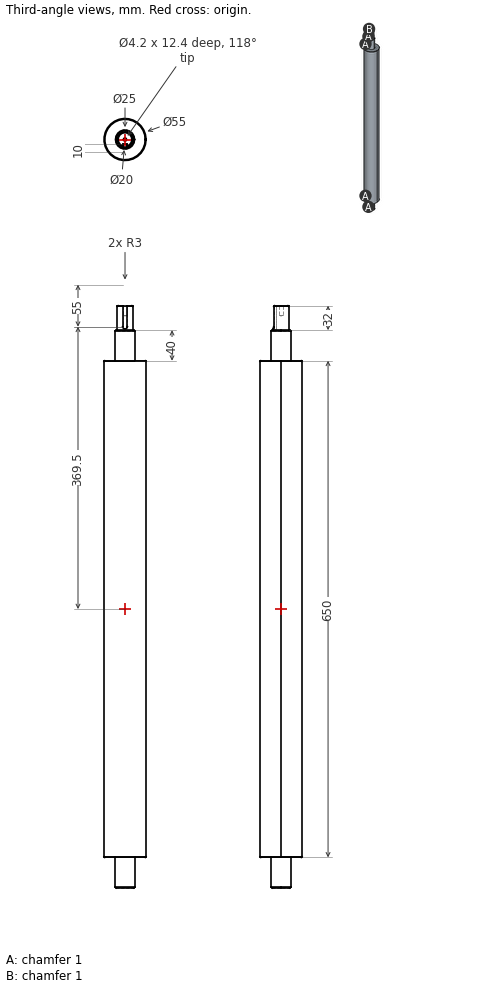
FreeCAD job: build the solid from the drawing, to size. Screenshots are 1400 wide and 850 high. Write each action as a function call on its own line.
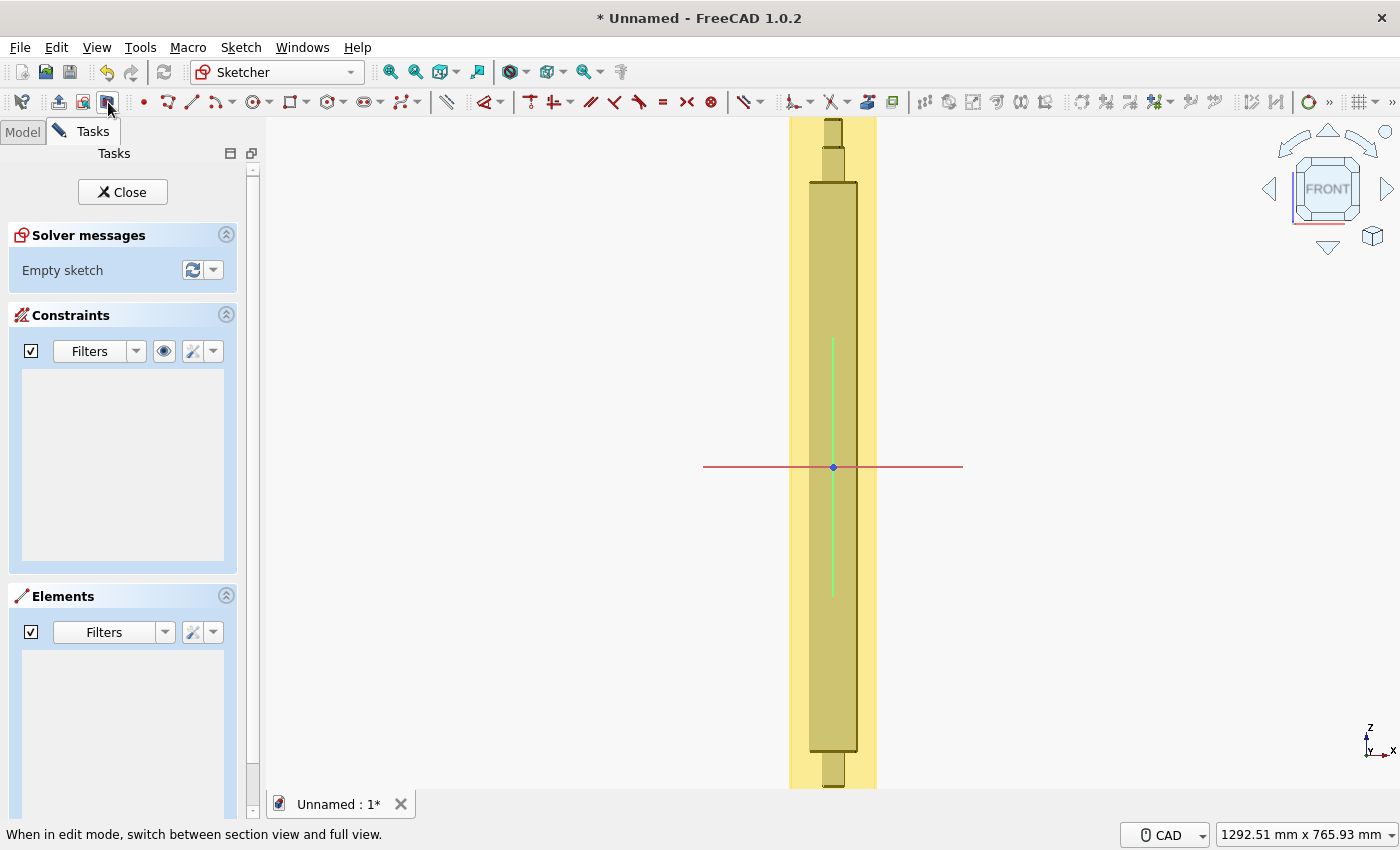
scroll(764, 453, down, 5)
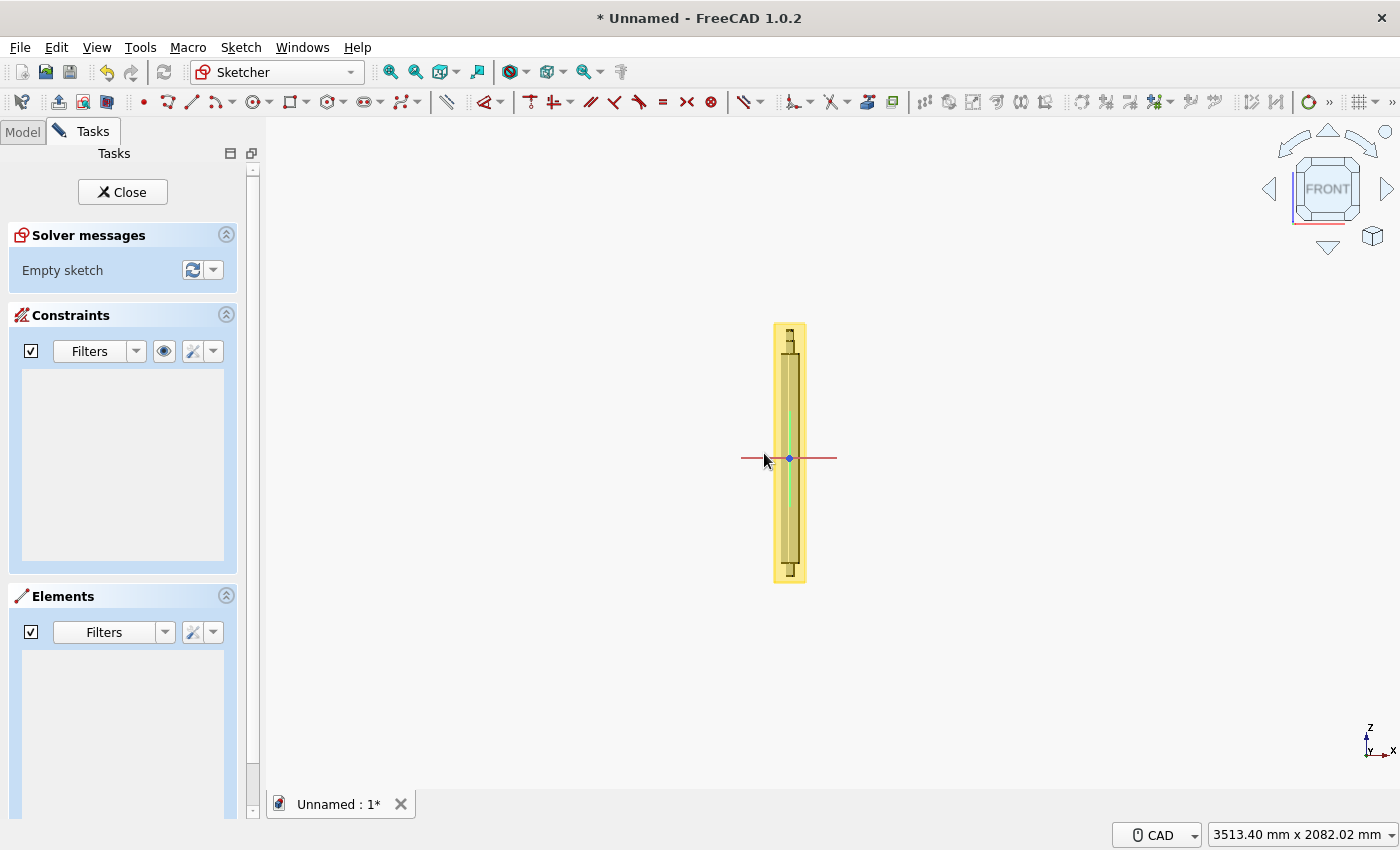
scroll(791, 324, up, 15)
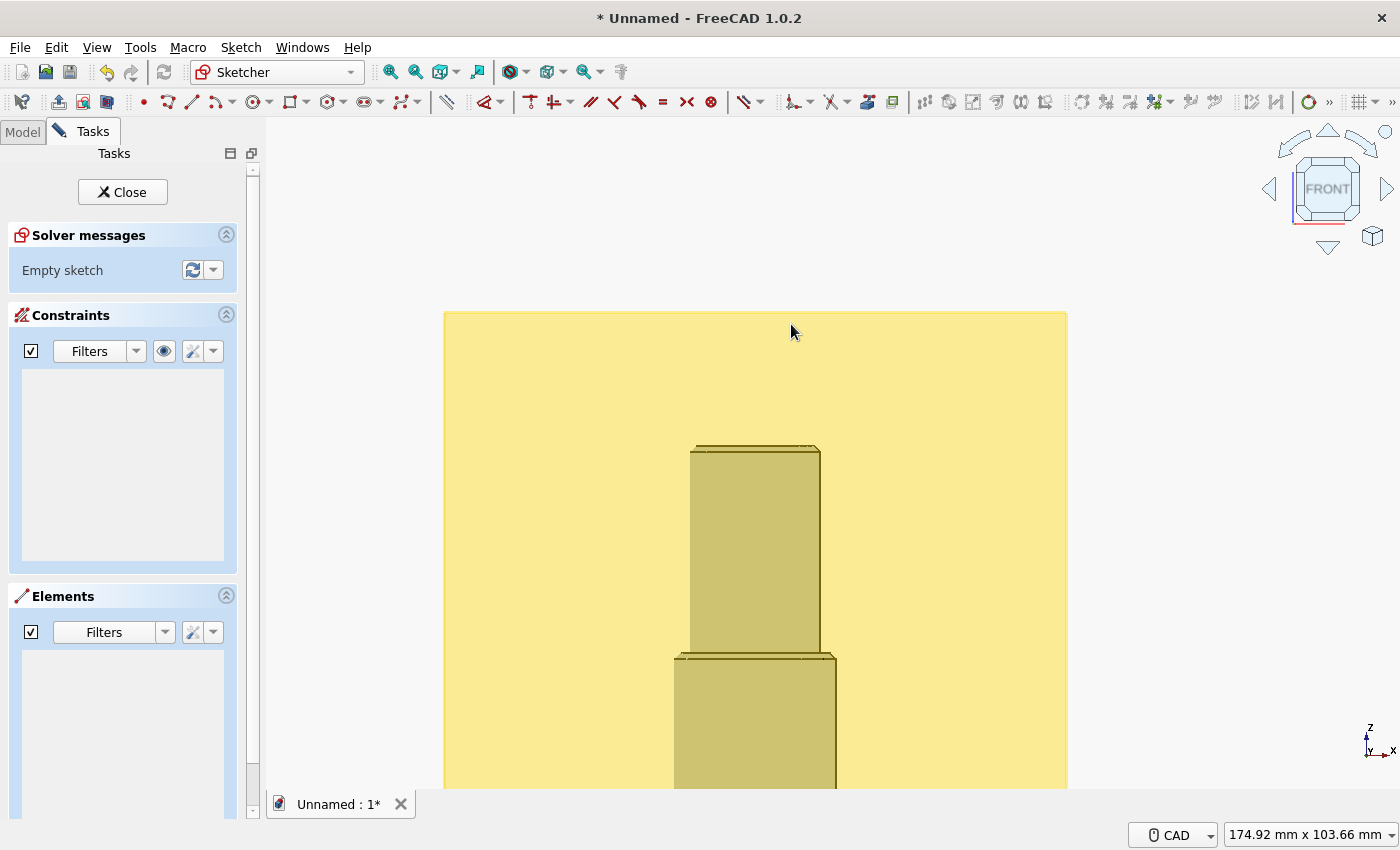
click(364, 102)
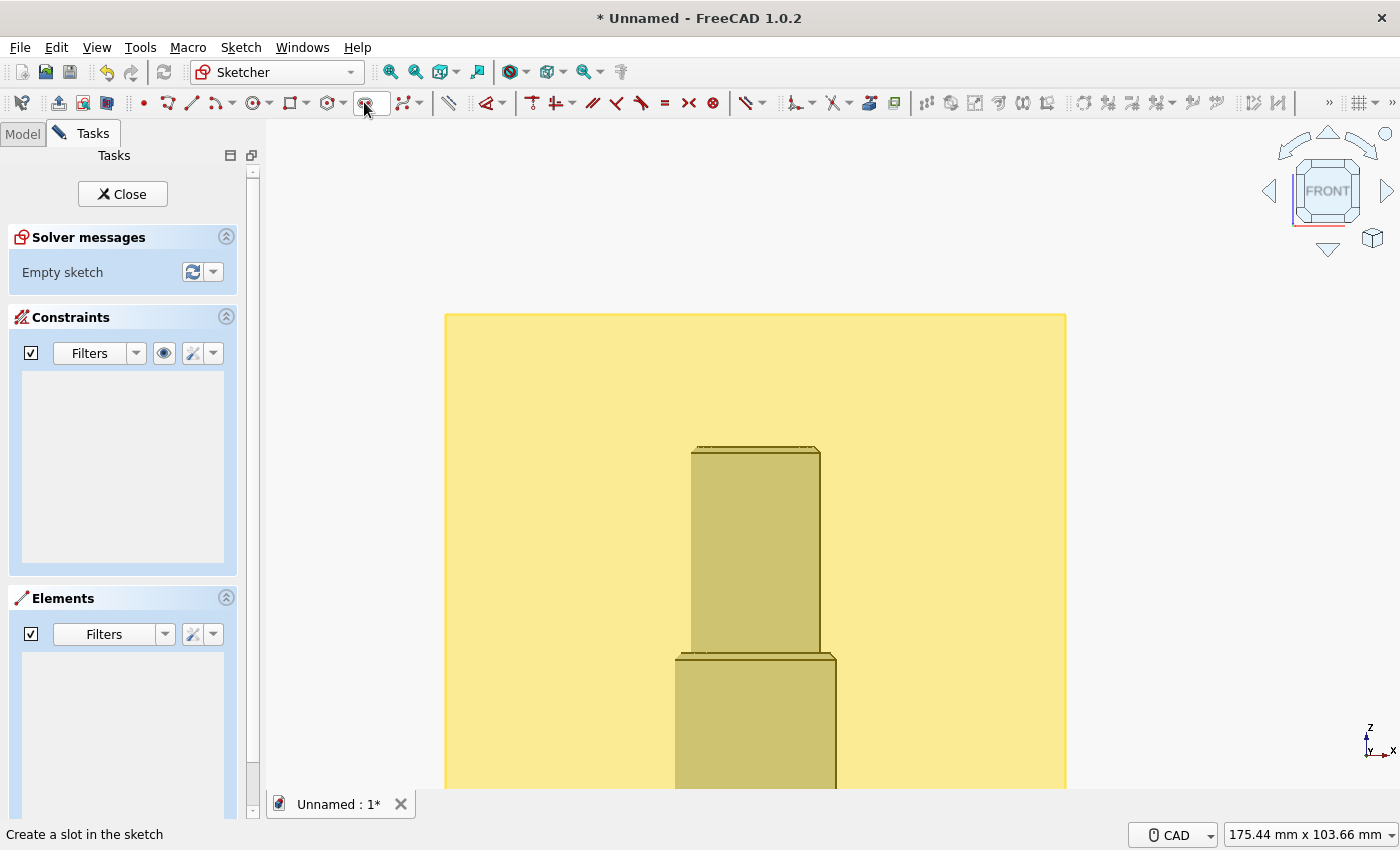
click(756, 624)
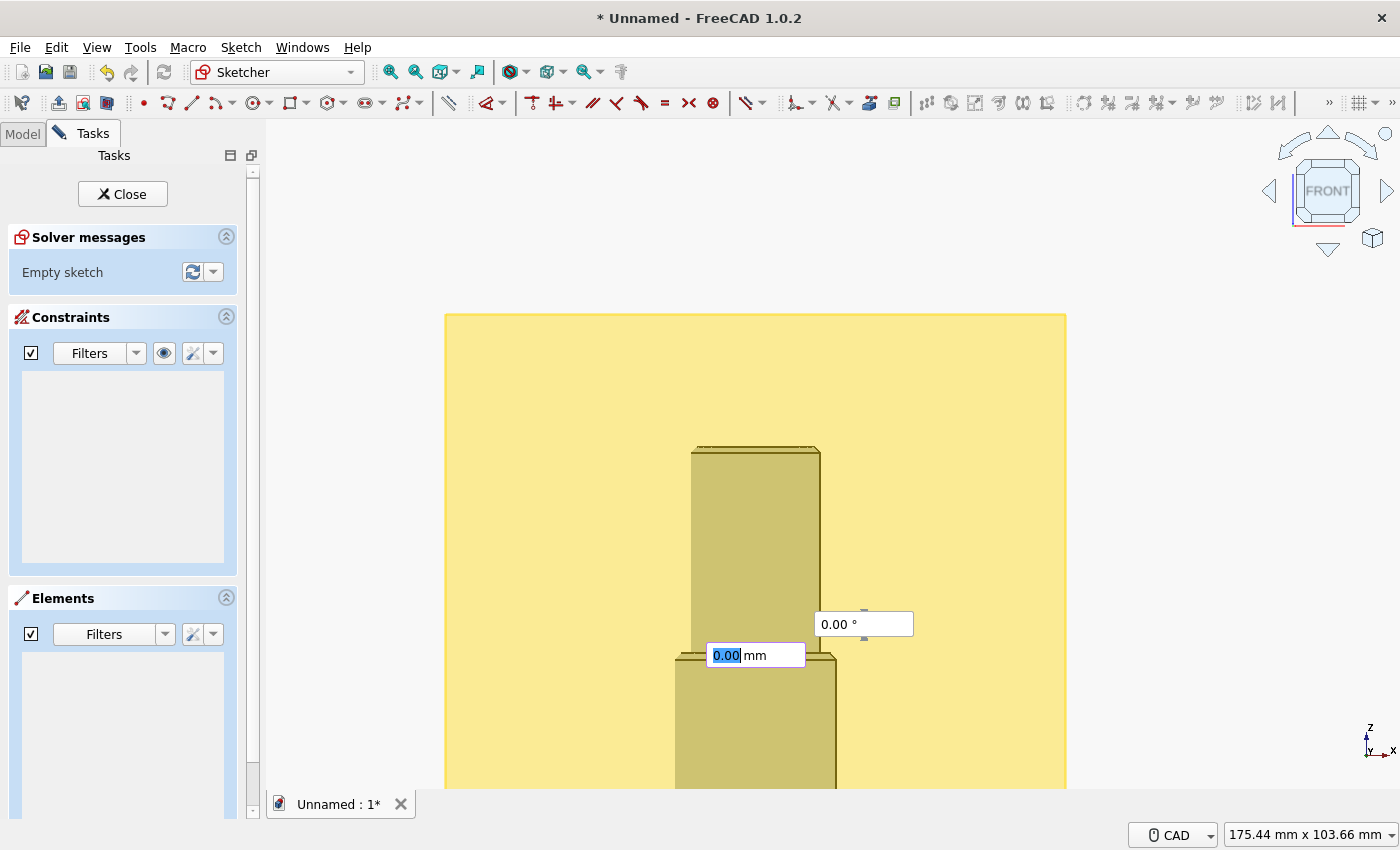
click(765, 269)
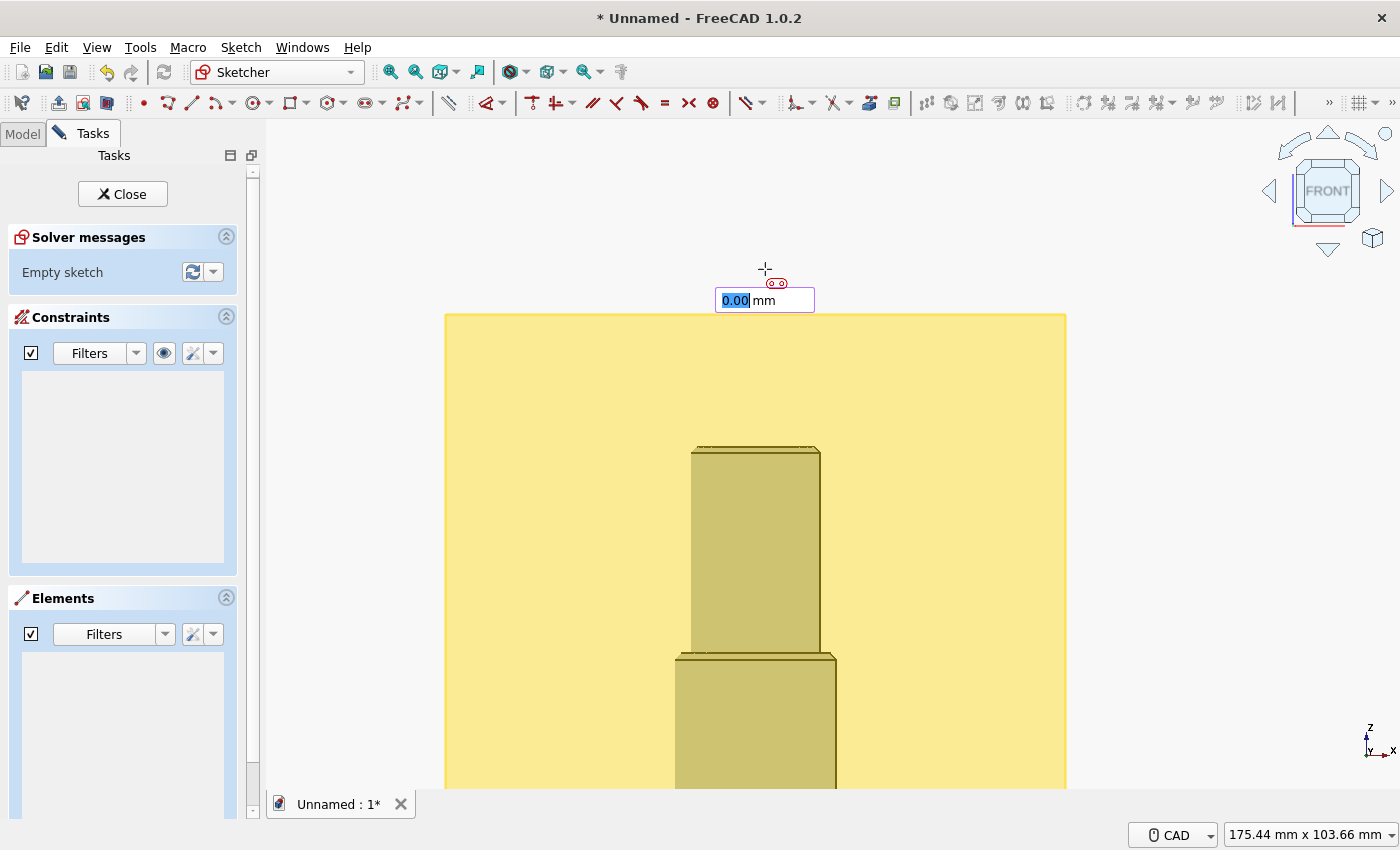
click(736, 447)
key(Escape)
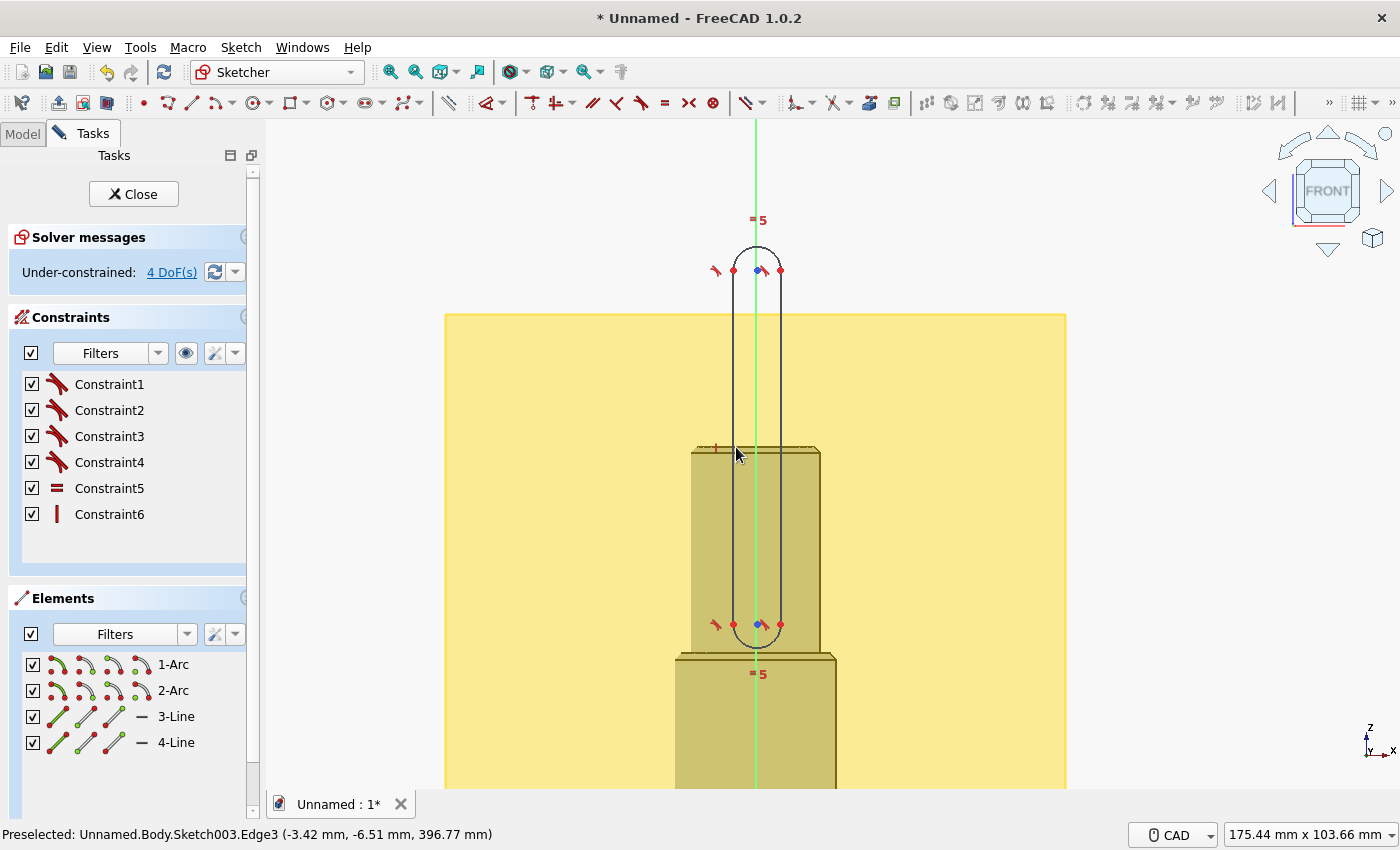
click(757, 624)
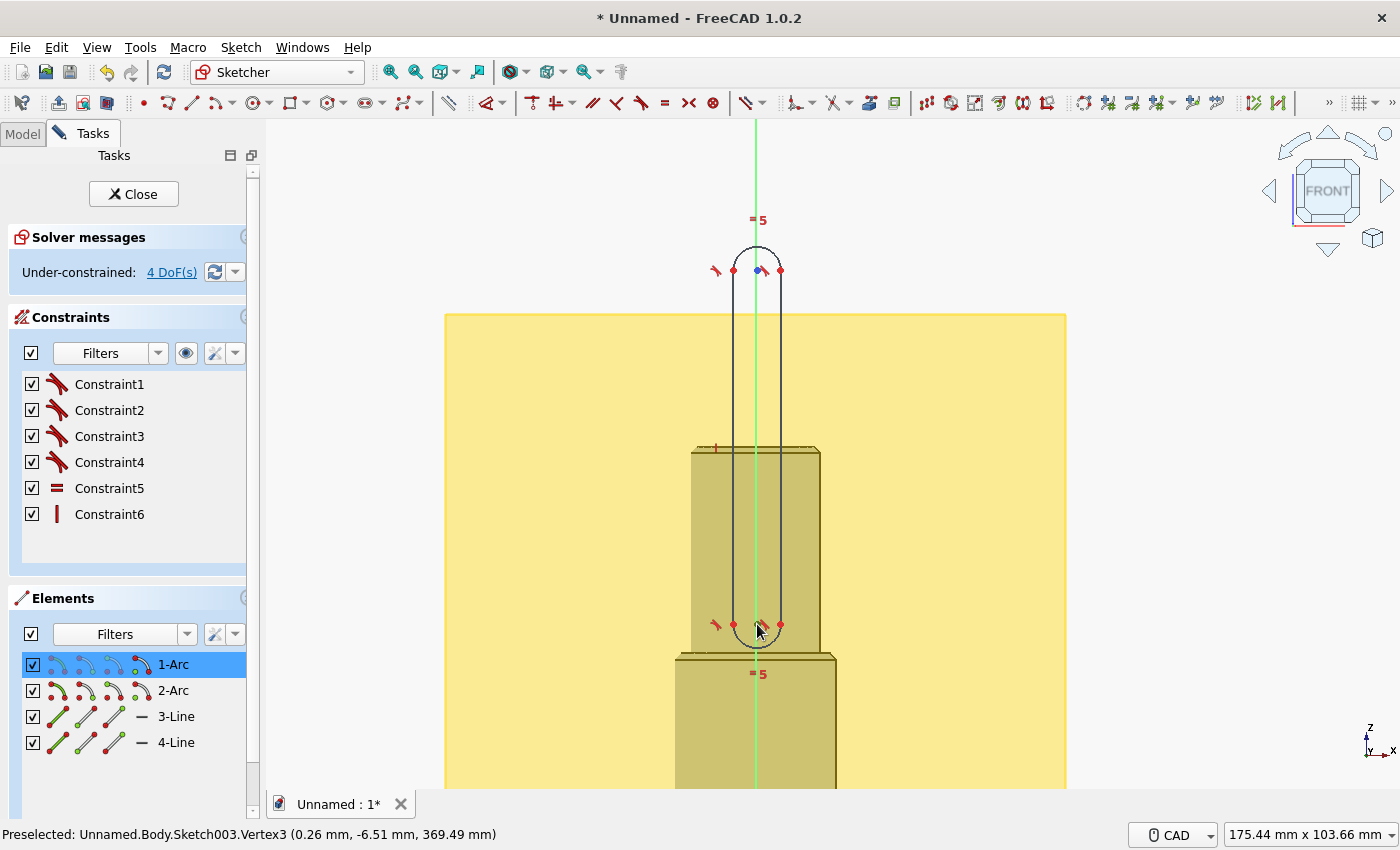
click(756, 717)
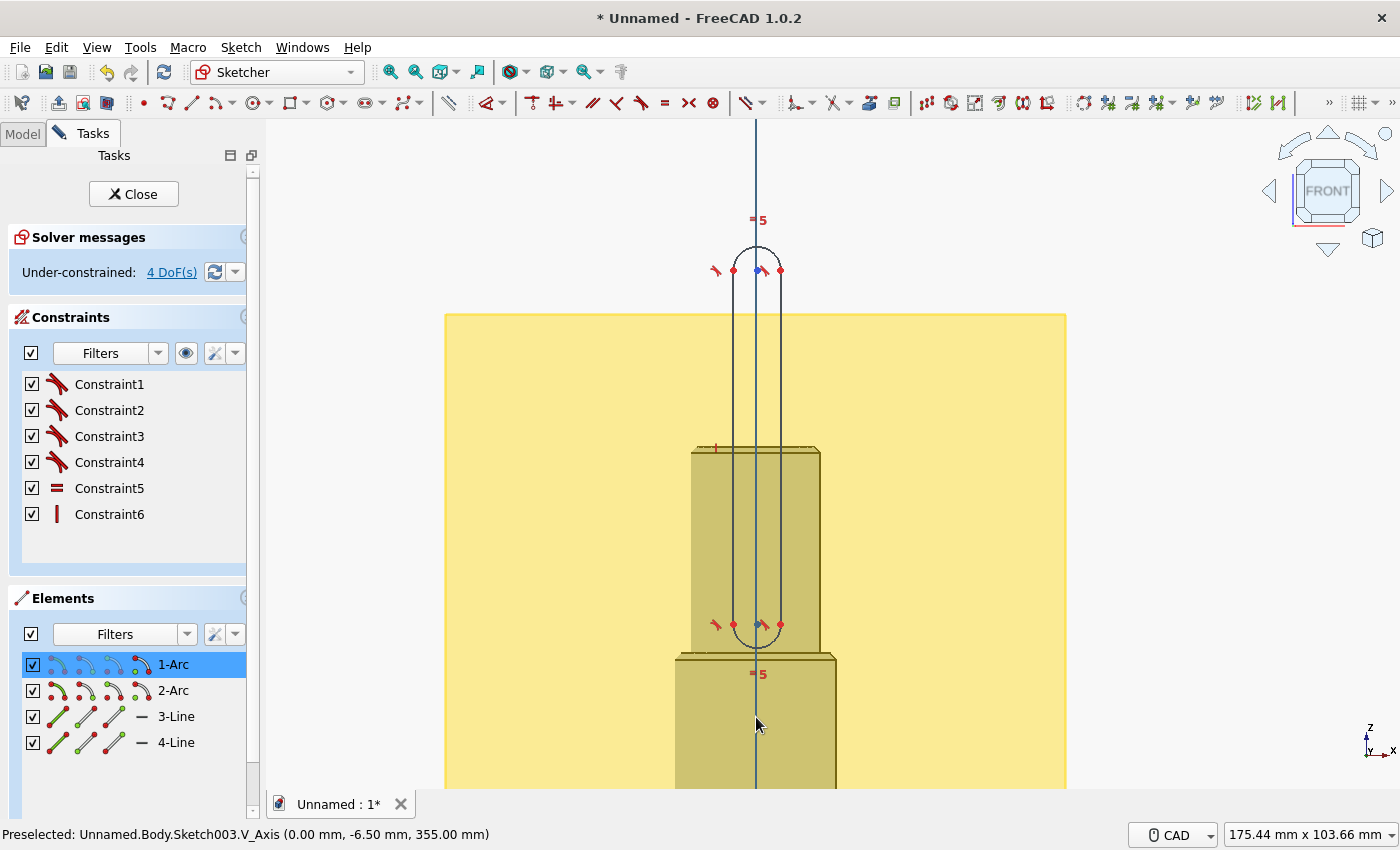
click(532, 104)